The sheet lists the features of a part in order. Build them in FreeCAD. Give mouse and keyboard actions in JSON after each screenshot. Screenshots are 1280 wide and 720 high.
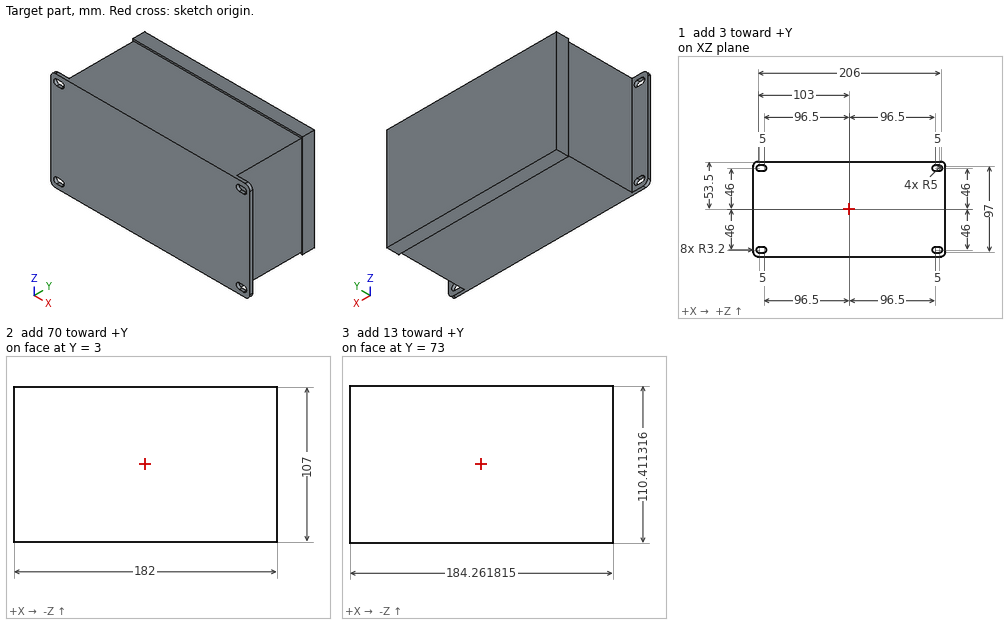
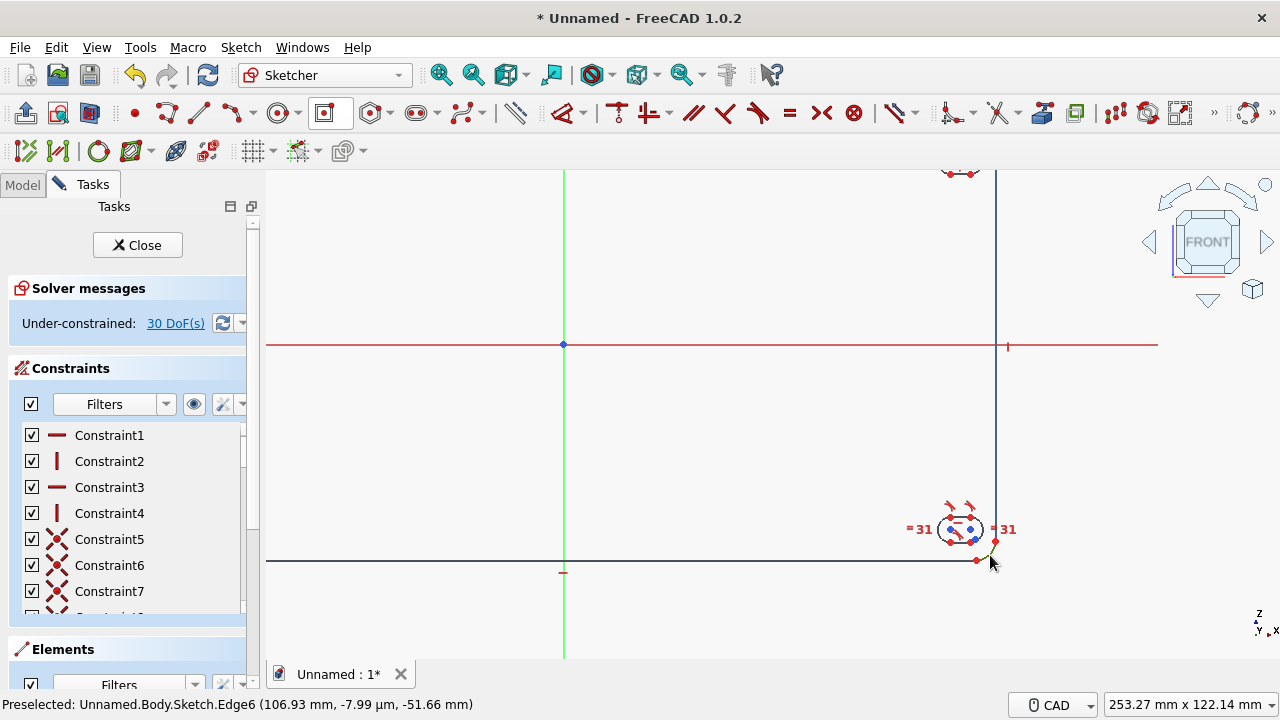
{"action": "left_click", "coordinate": [758, 114]}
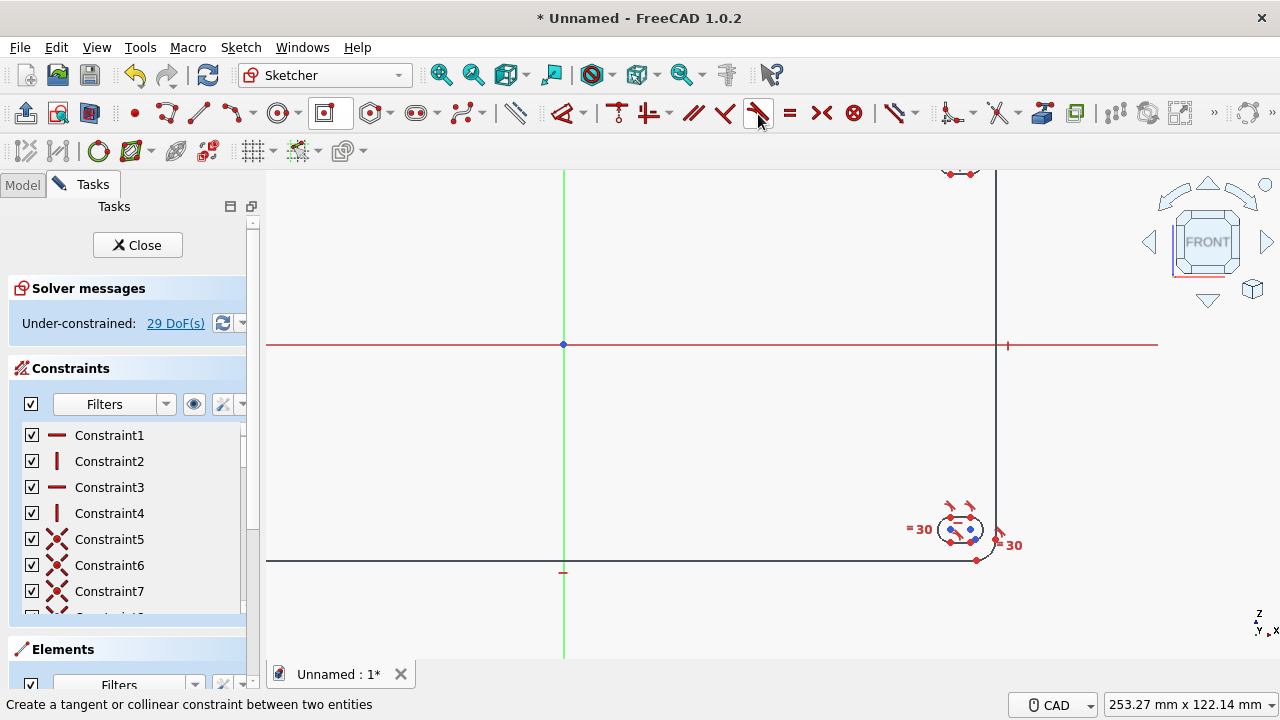
{"action": "left_click", "coordinate": [729, 561]}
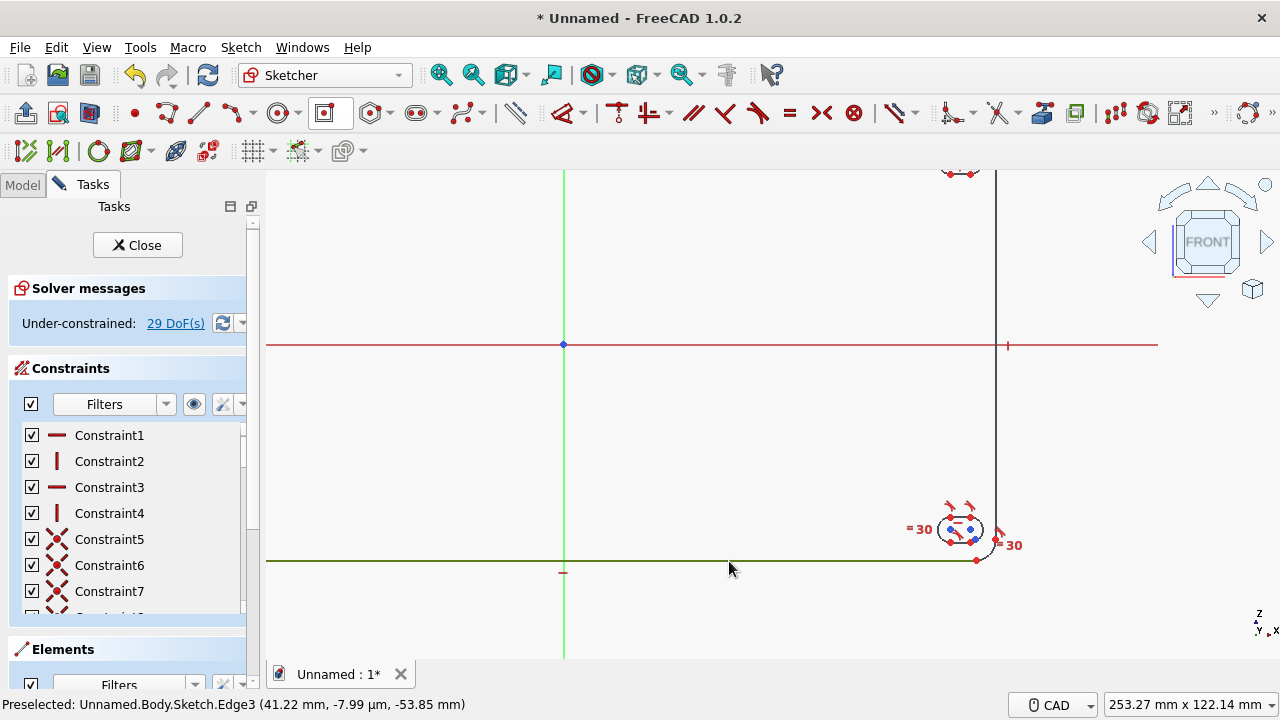
{"action": "scroll", "coordinate": [985, 558], "scroll_direction": "up", "scroll_amount": 2}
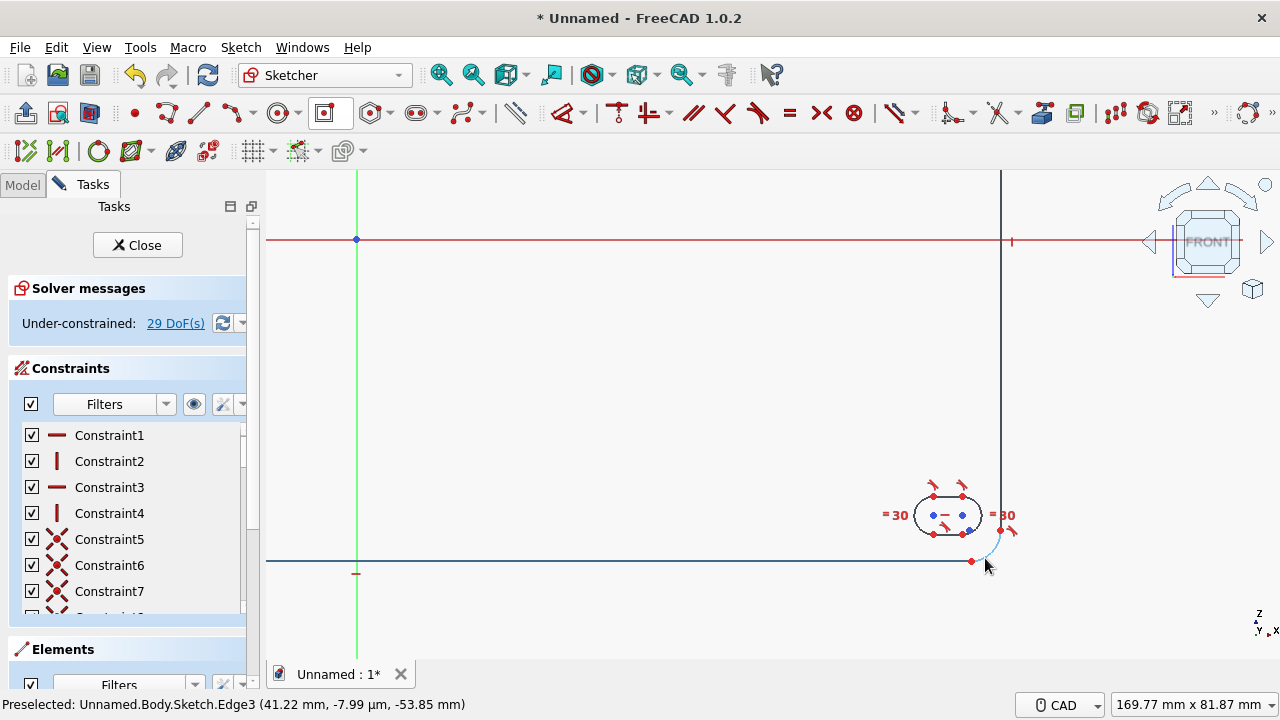
{"action": "left_click", "coordinate": [985, 557]}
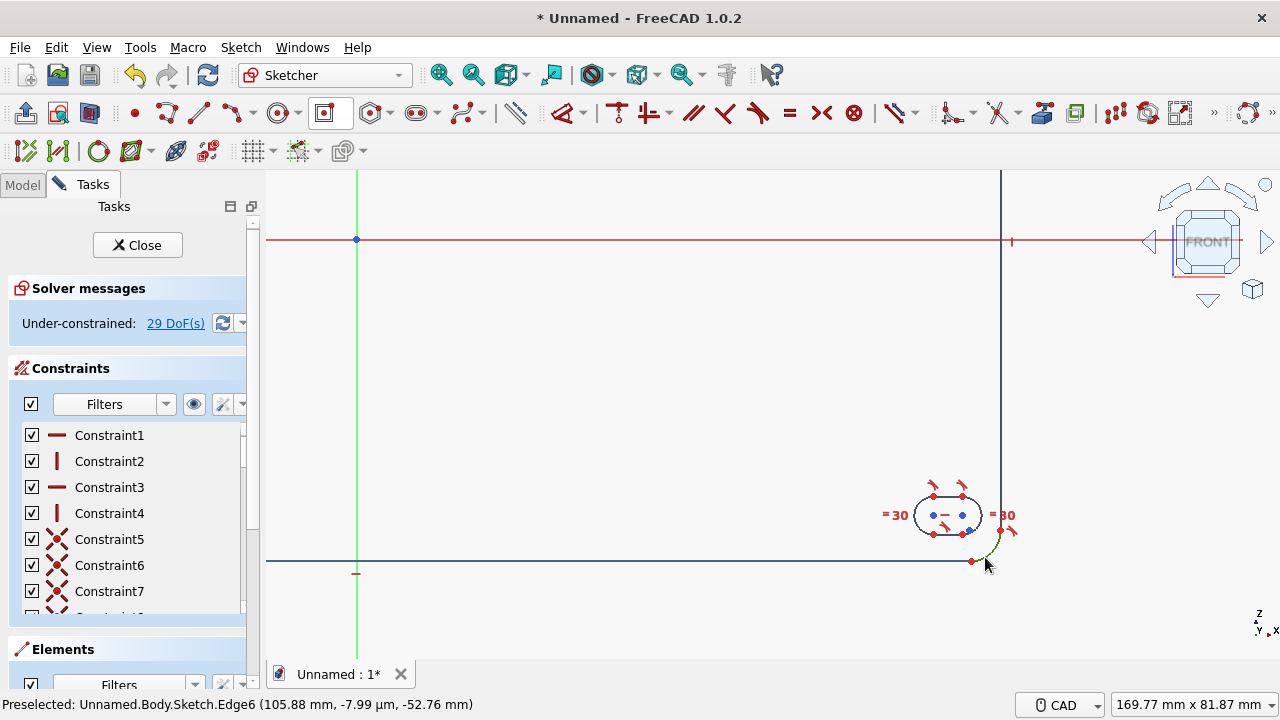
{"action": "left_click", "coordinate": [758, 114]}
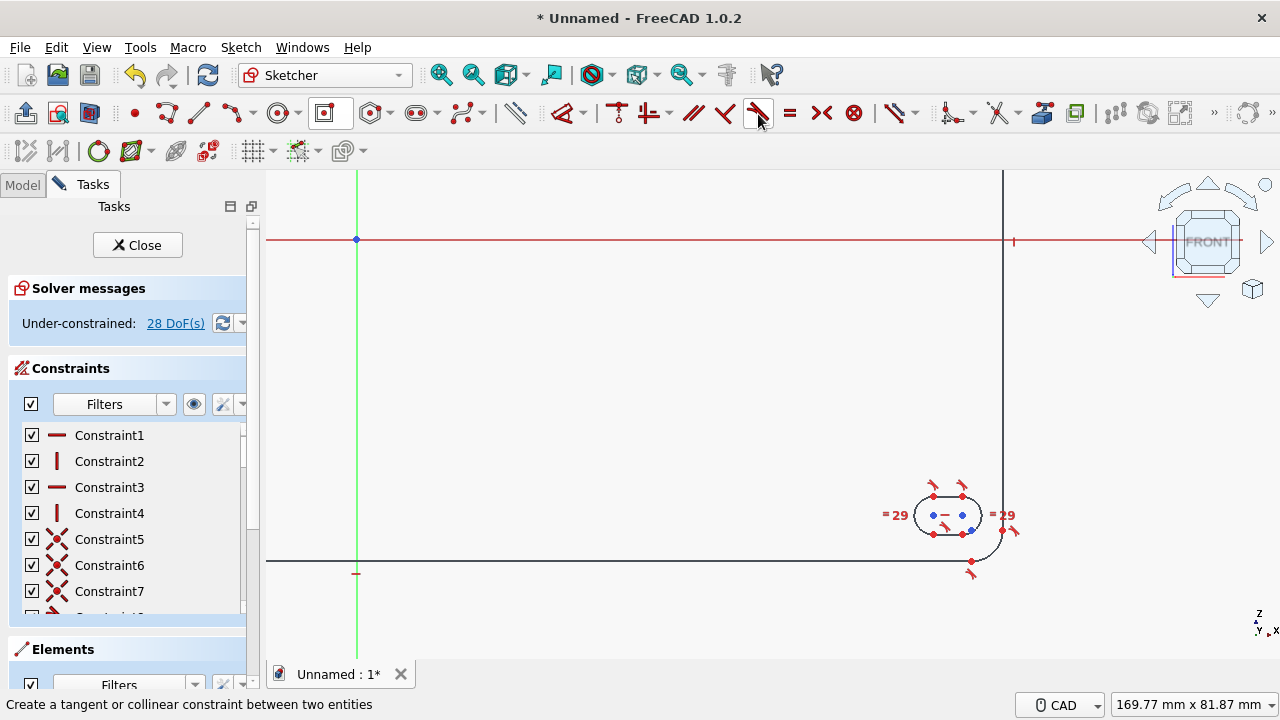
{"action": "left_click", "coordinate": [603, 561]}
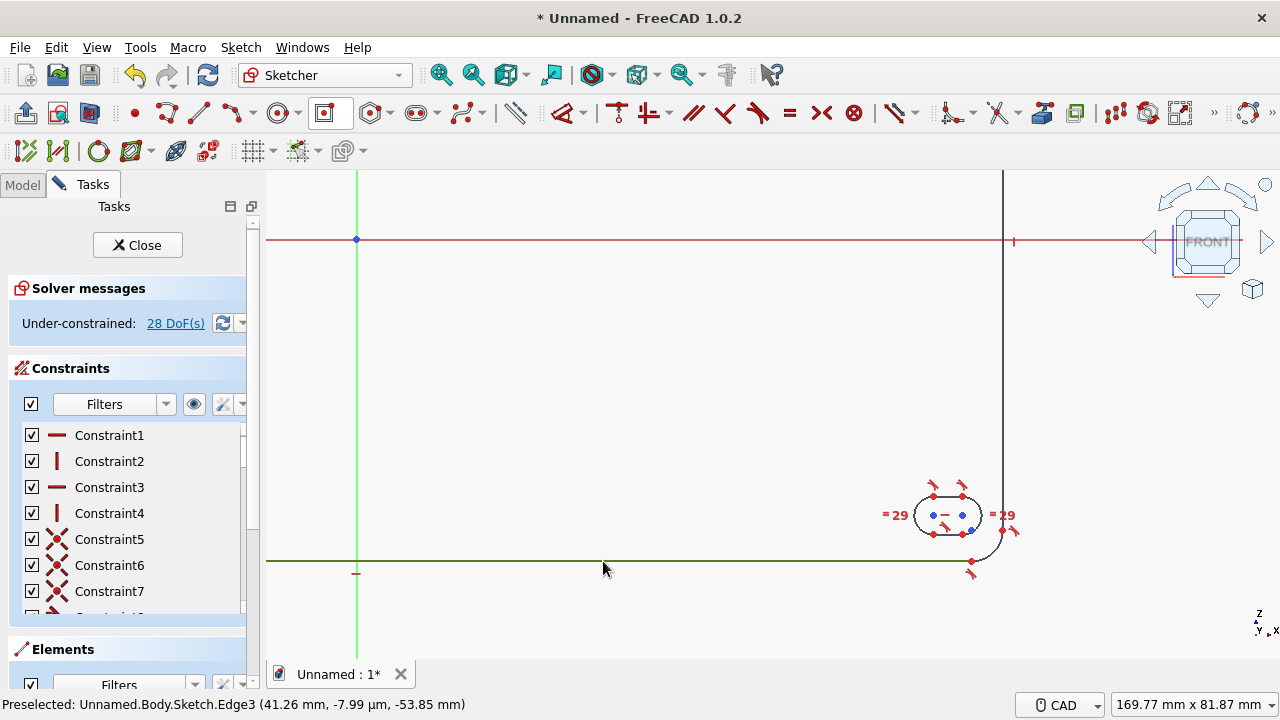
{"action": "scroll", "coordinate": [988, 557], "scroll_direction": "down", "scroll_amount": 4}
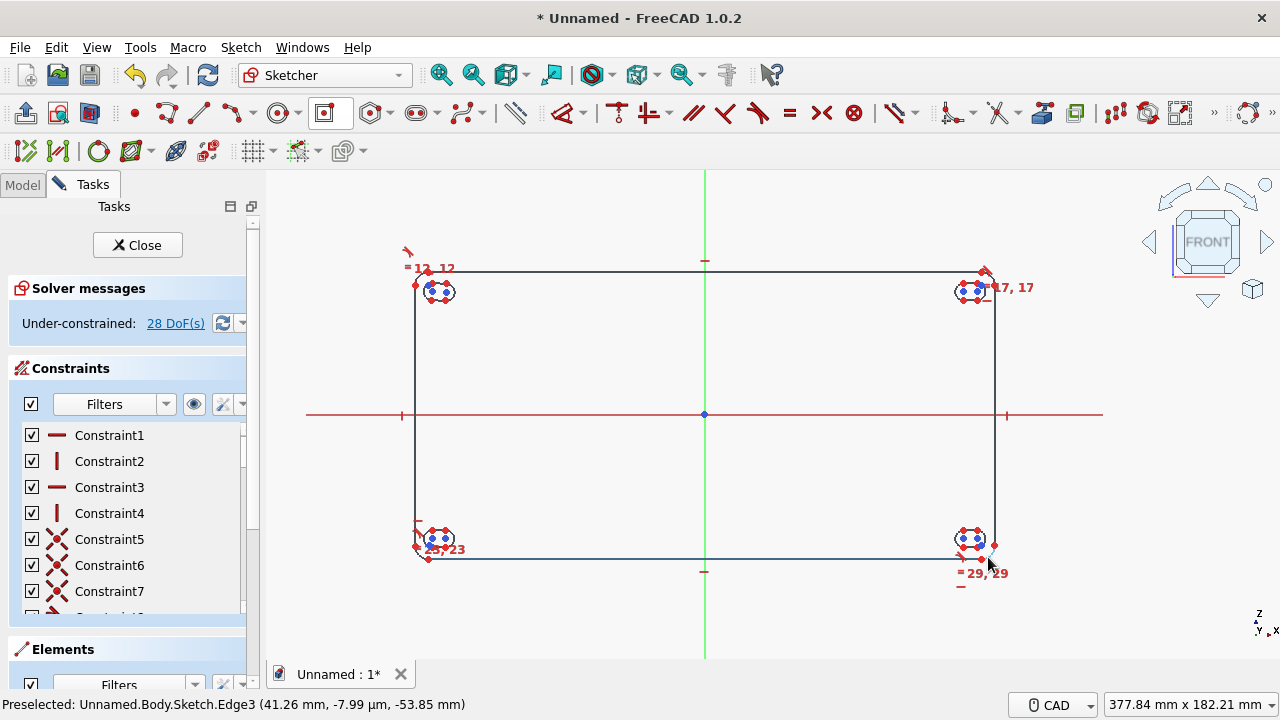
{"action": "scroll", "coordinate": [417, 552], "scroll_direction": "up", "scroll_amount": 5}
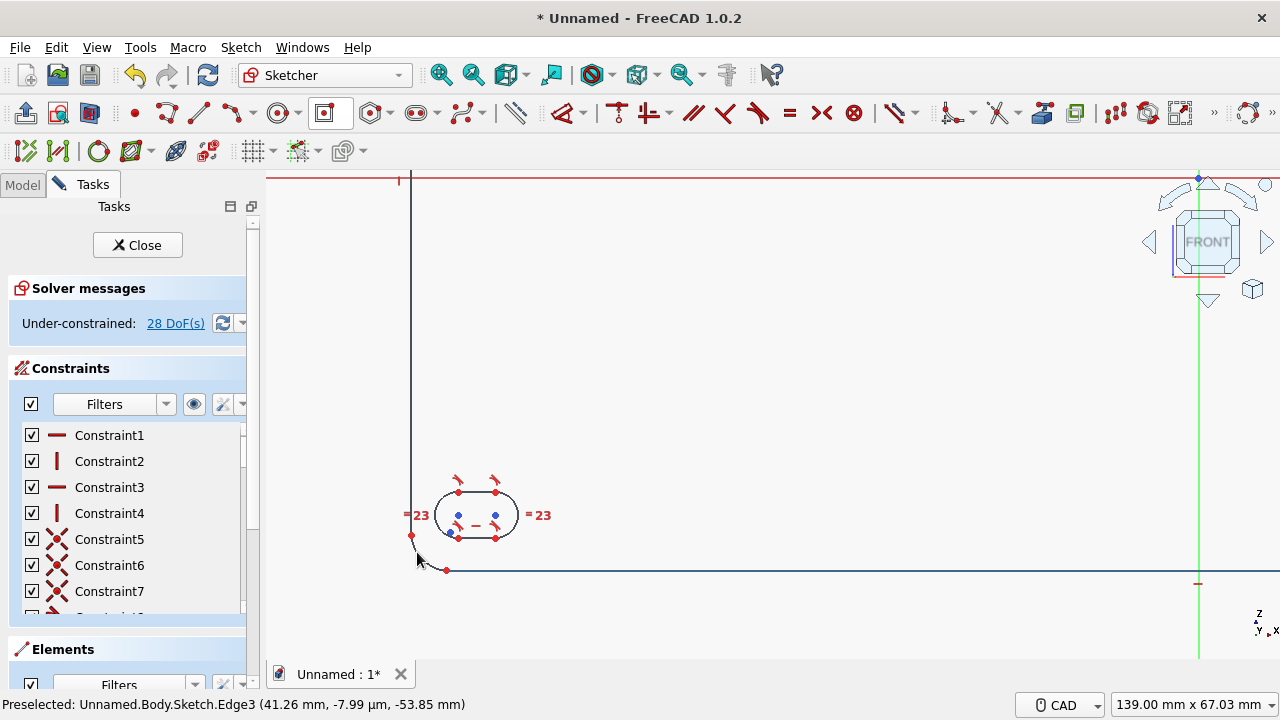
{"action": "left_click", "coordinate": [416, 551]}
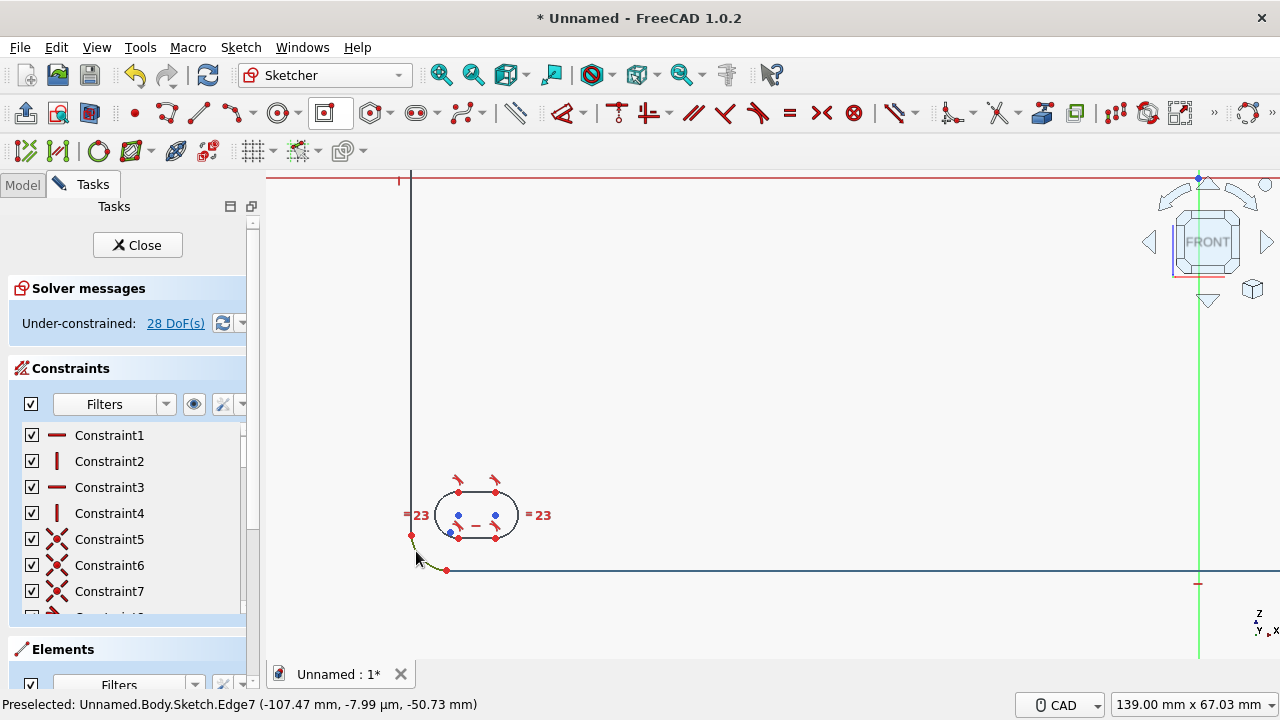
{"action": "left_click", "coordinate": [758, 114]}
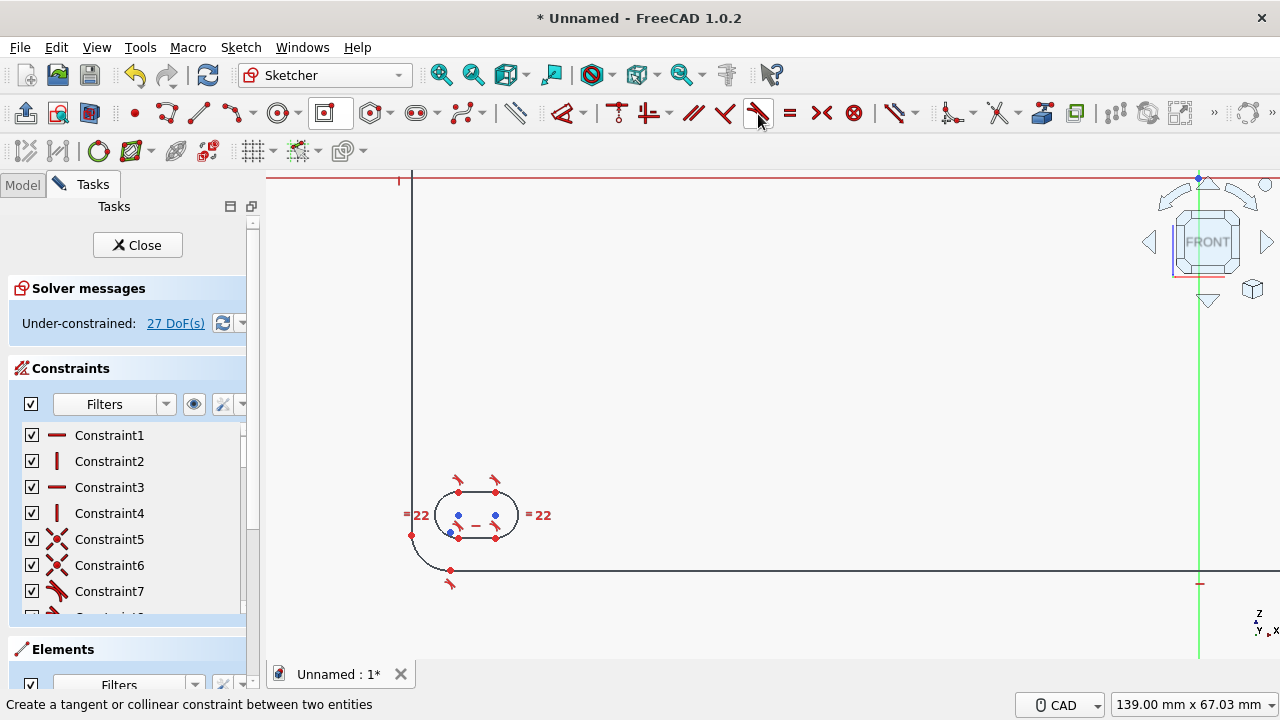
{"action": "left_click", "coordinate": [412, 323]}